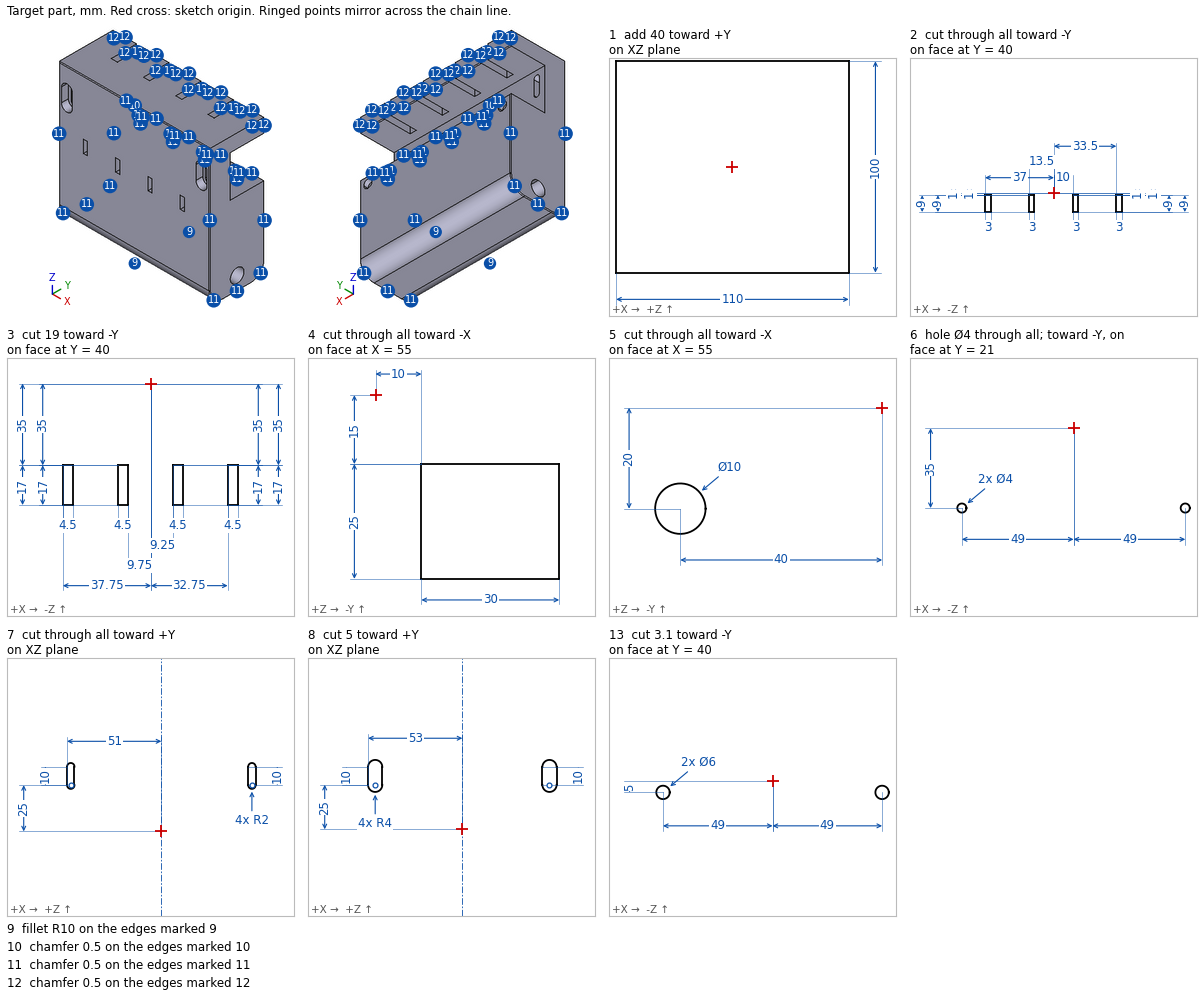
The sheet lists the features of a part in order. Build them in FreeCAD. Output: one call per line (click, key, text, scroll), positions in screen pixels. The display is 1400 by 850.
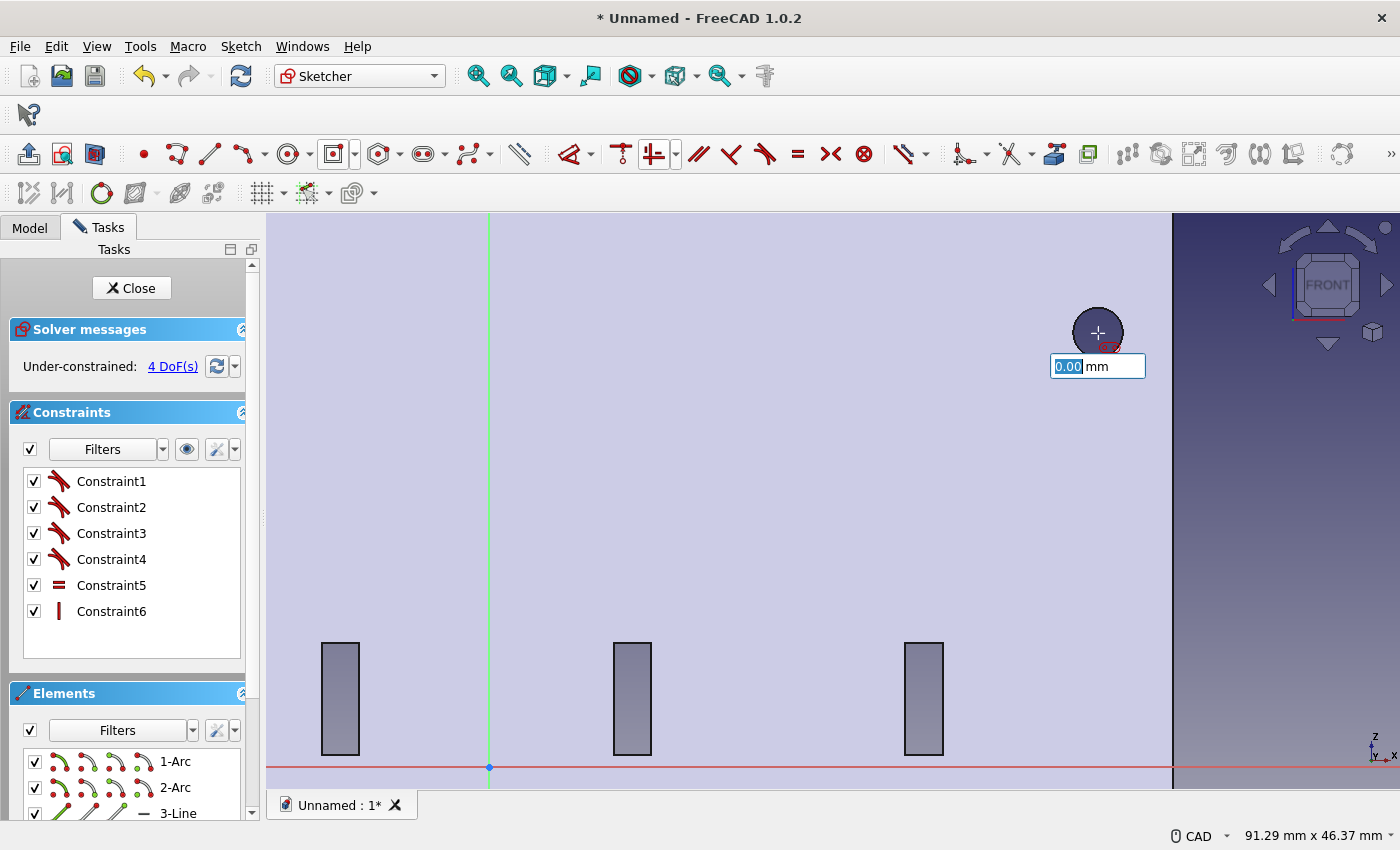
click(1073, 395)
key(Escape)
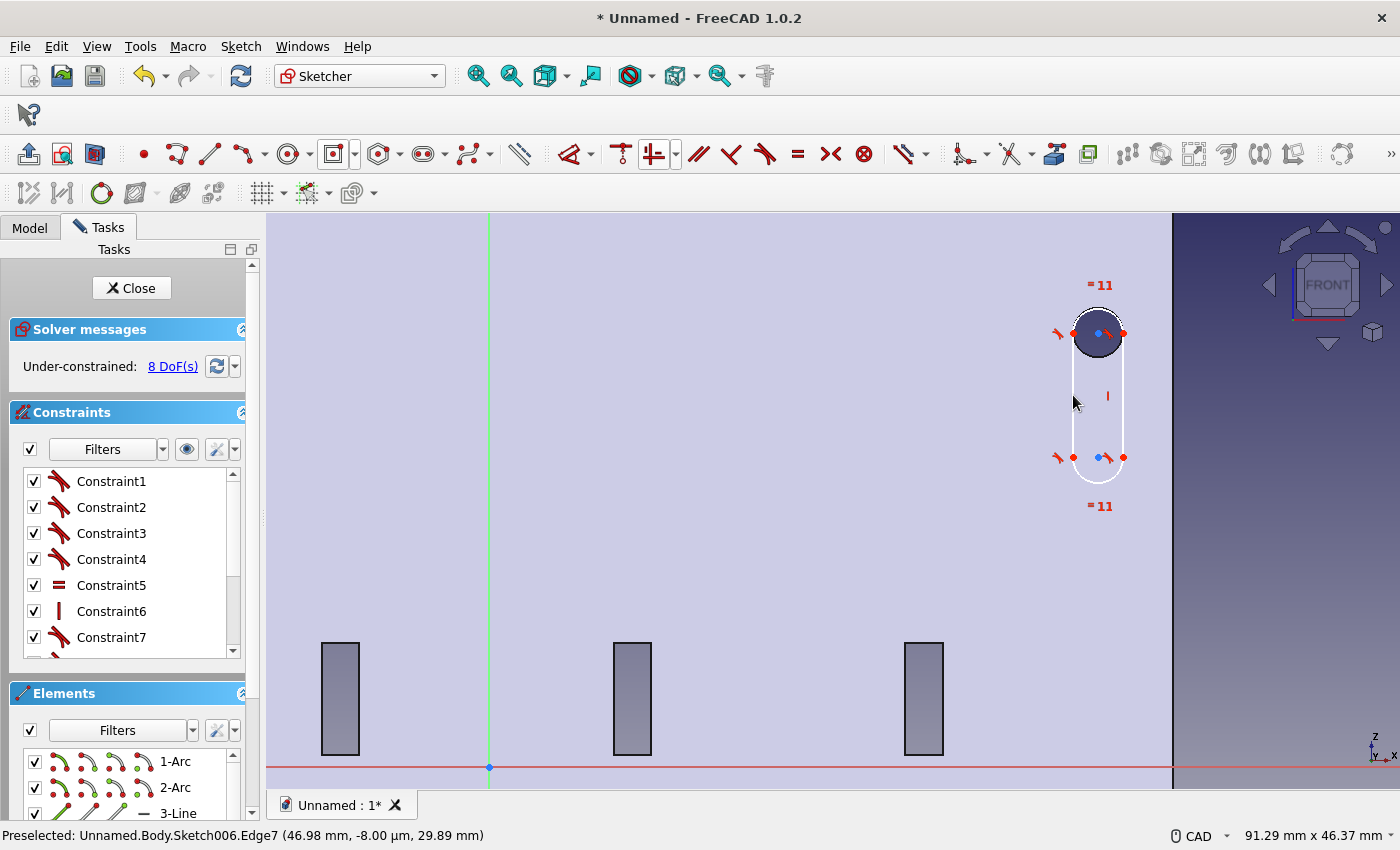
scroll(1099, 457, down, 3)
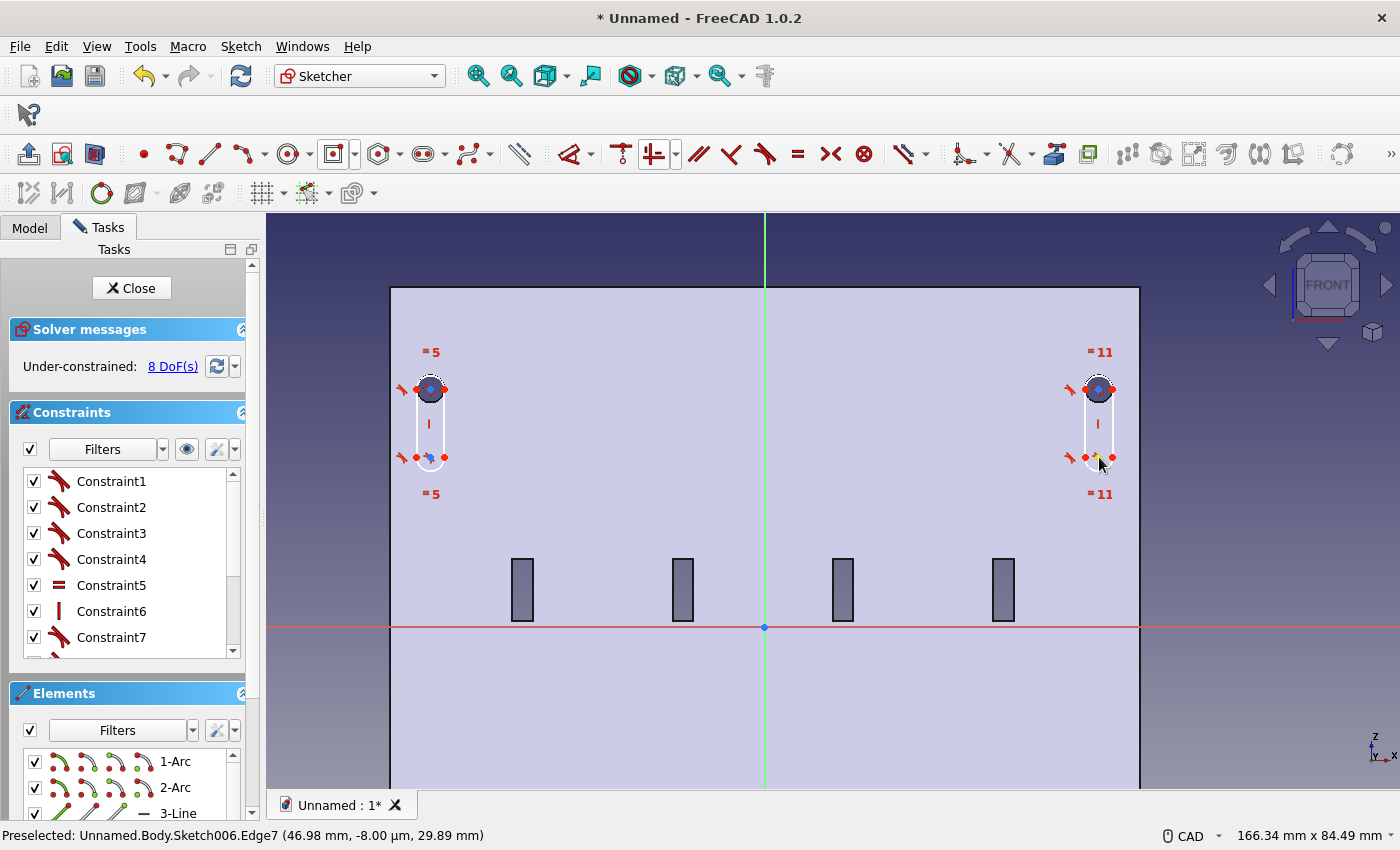
click(422, 469)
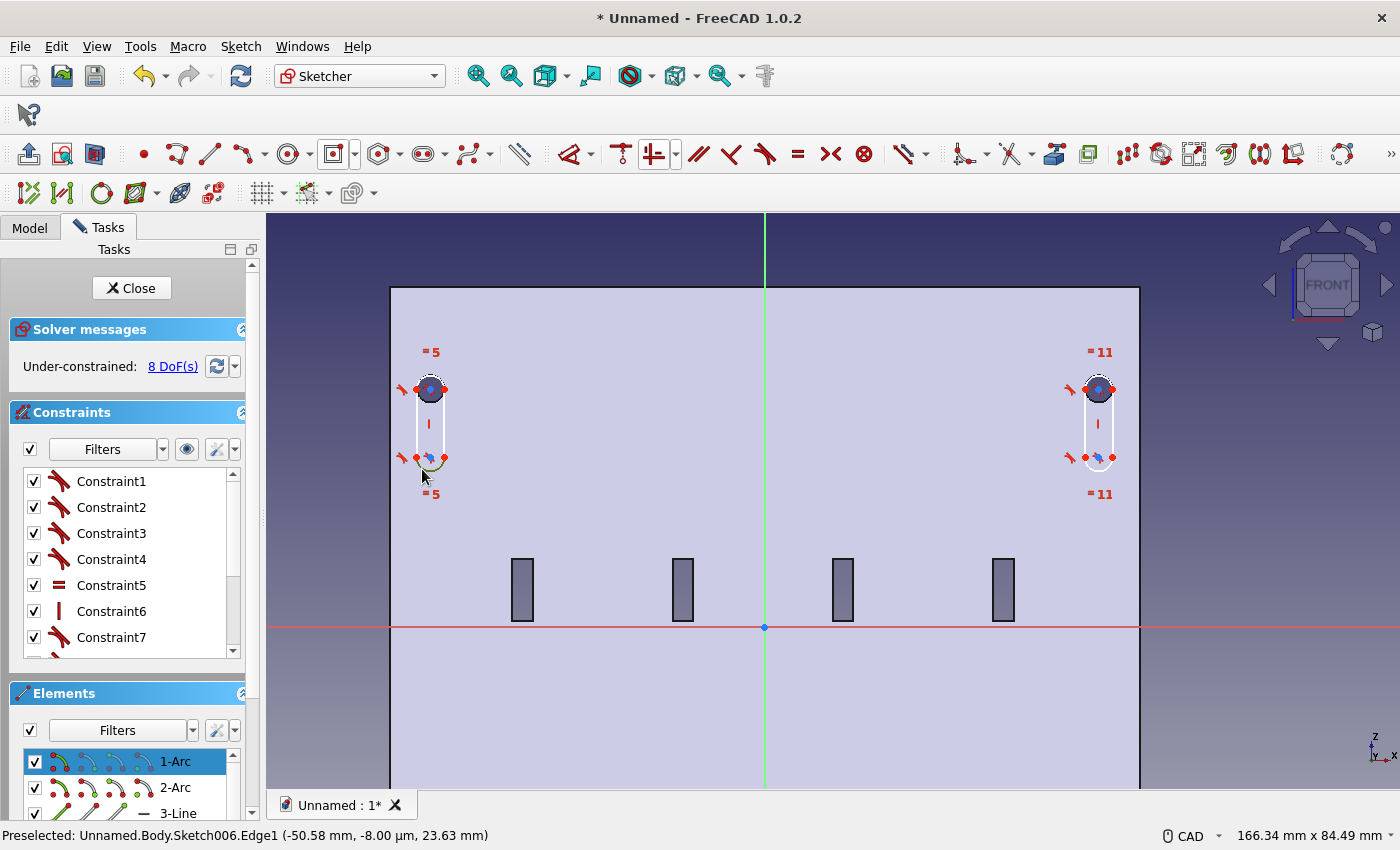
click(1091, 469)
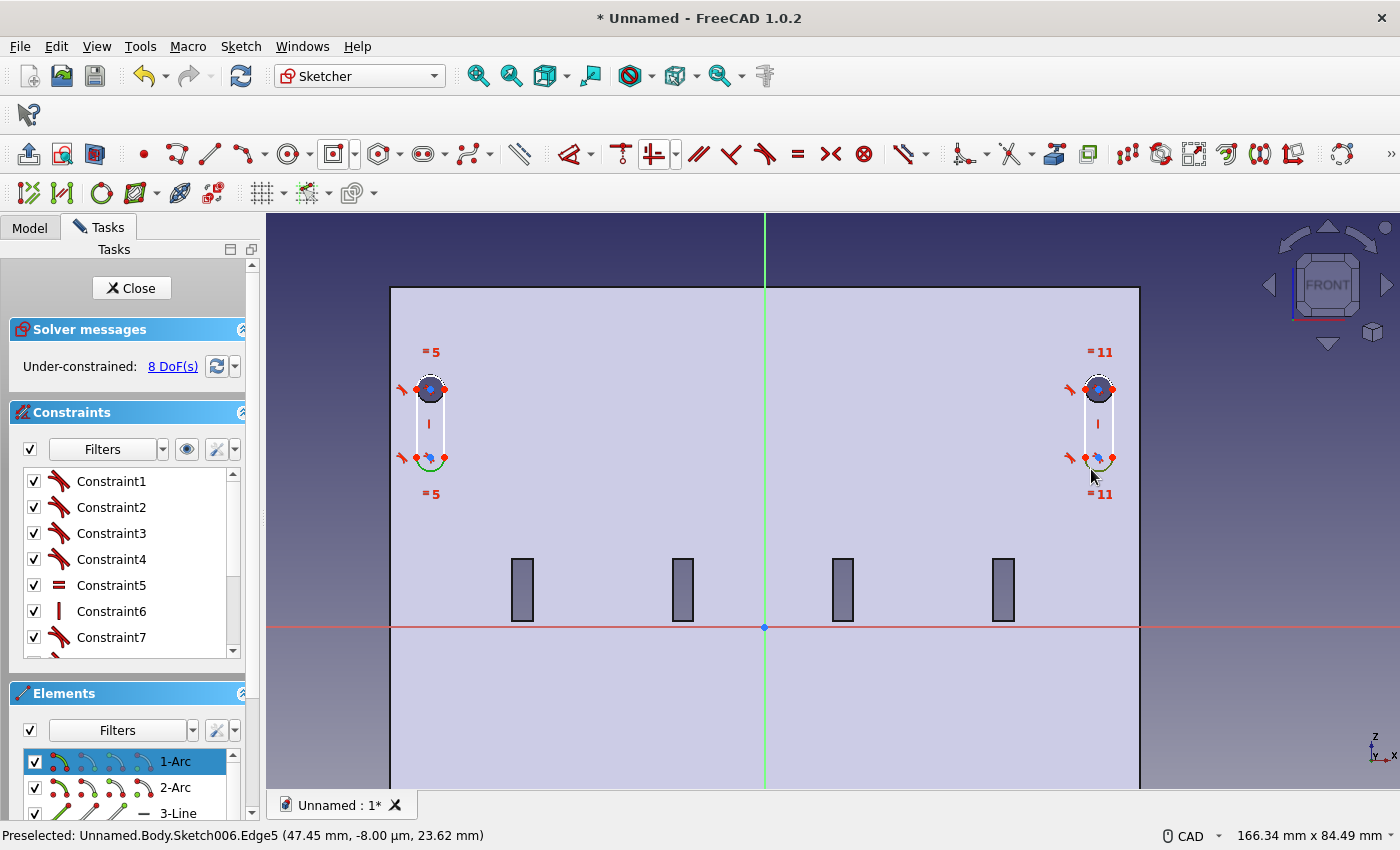
click(798, 154)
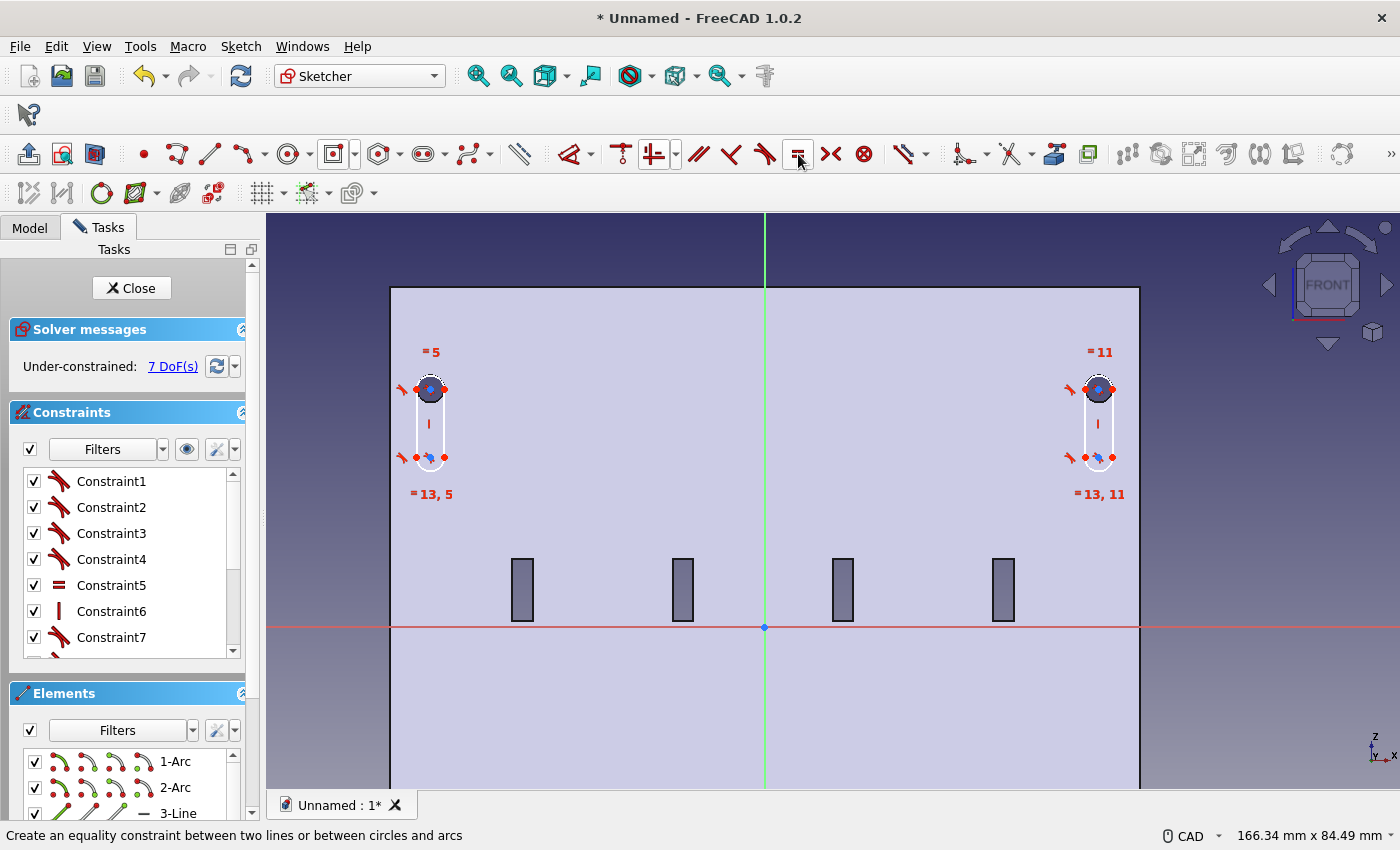
click(431, 458)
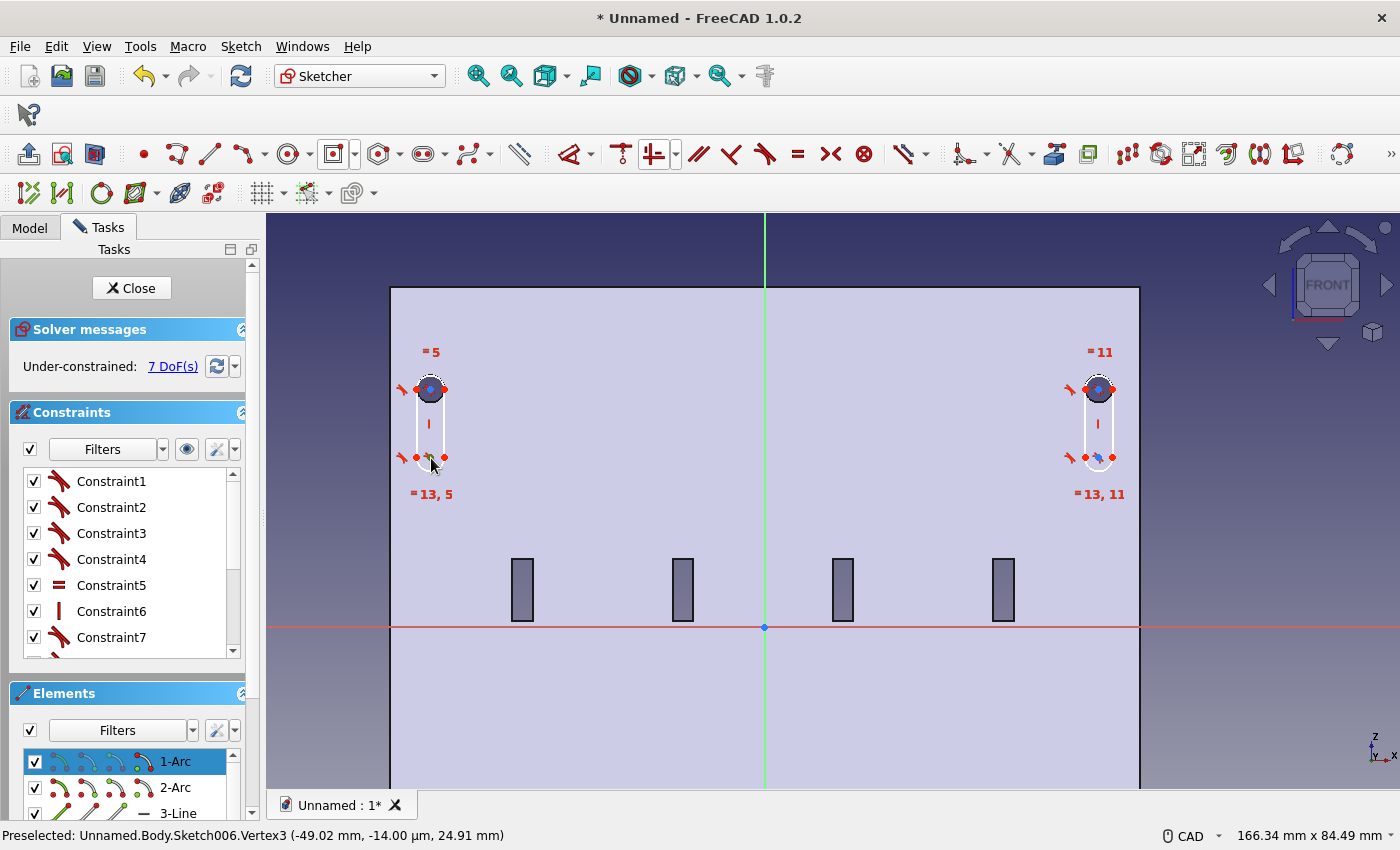
click(1099, 458)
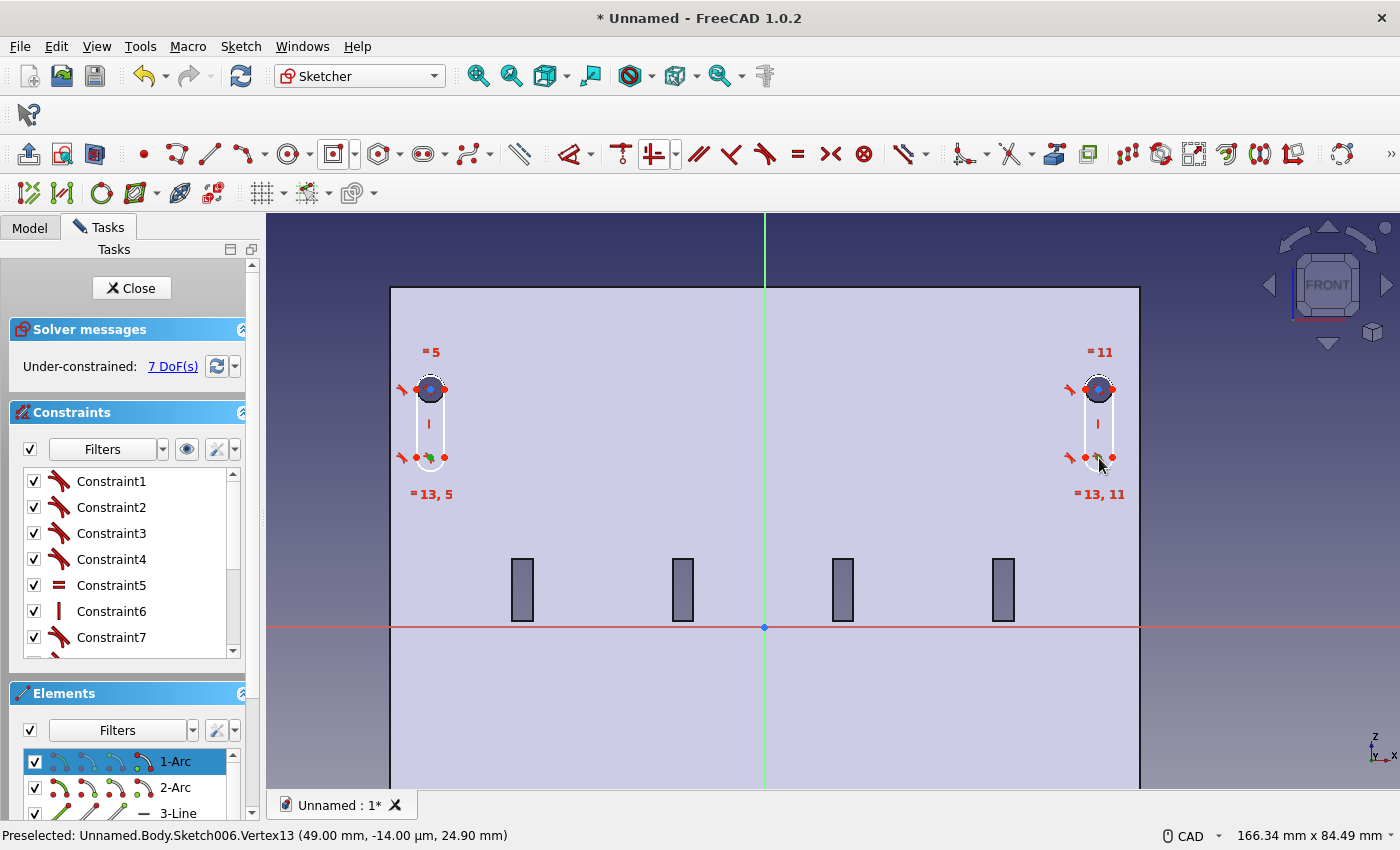
click(765, 724)